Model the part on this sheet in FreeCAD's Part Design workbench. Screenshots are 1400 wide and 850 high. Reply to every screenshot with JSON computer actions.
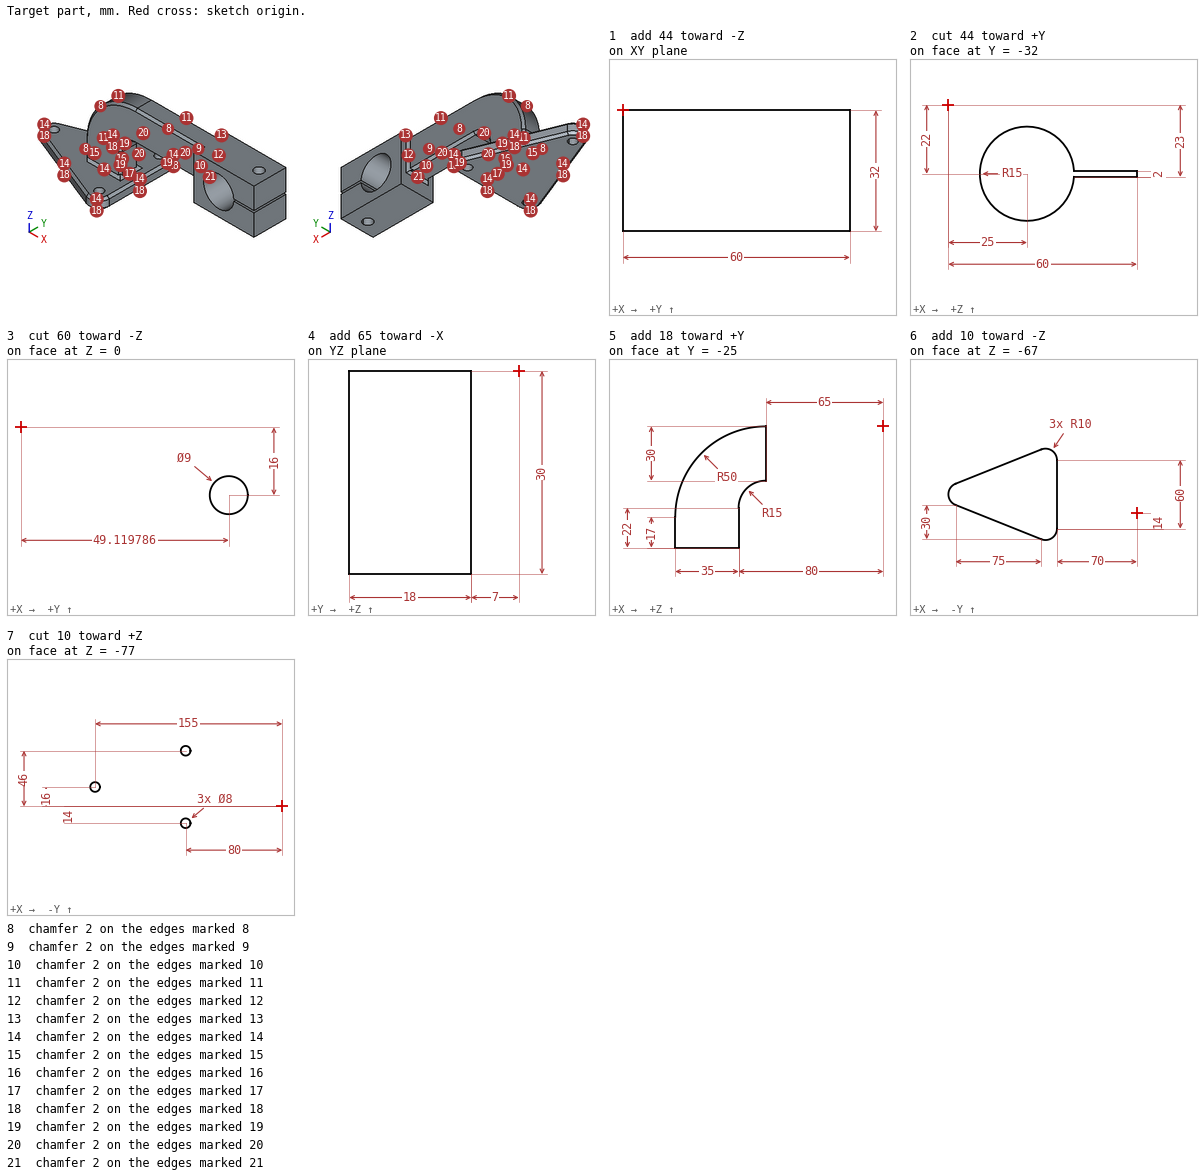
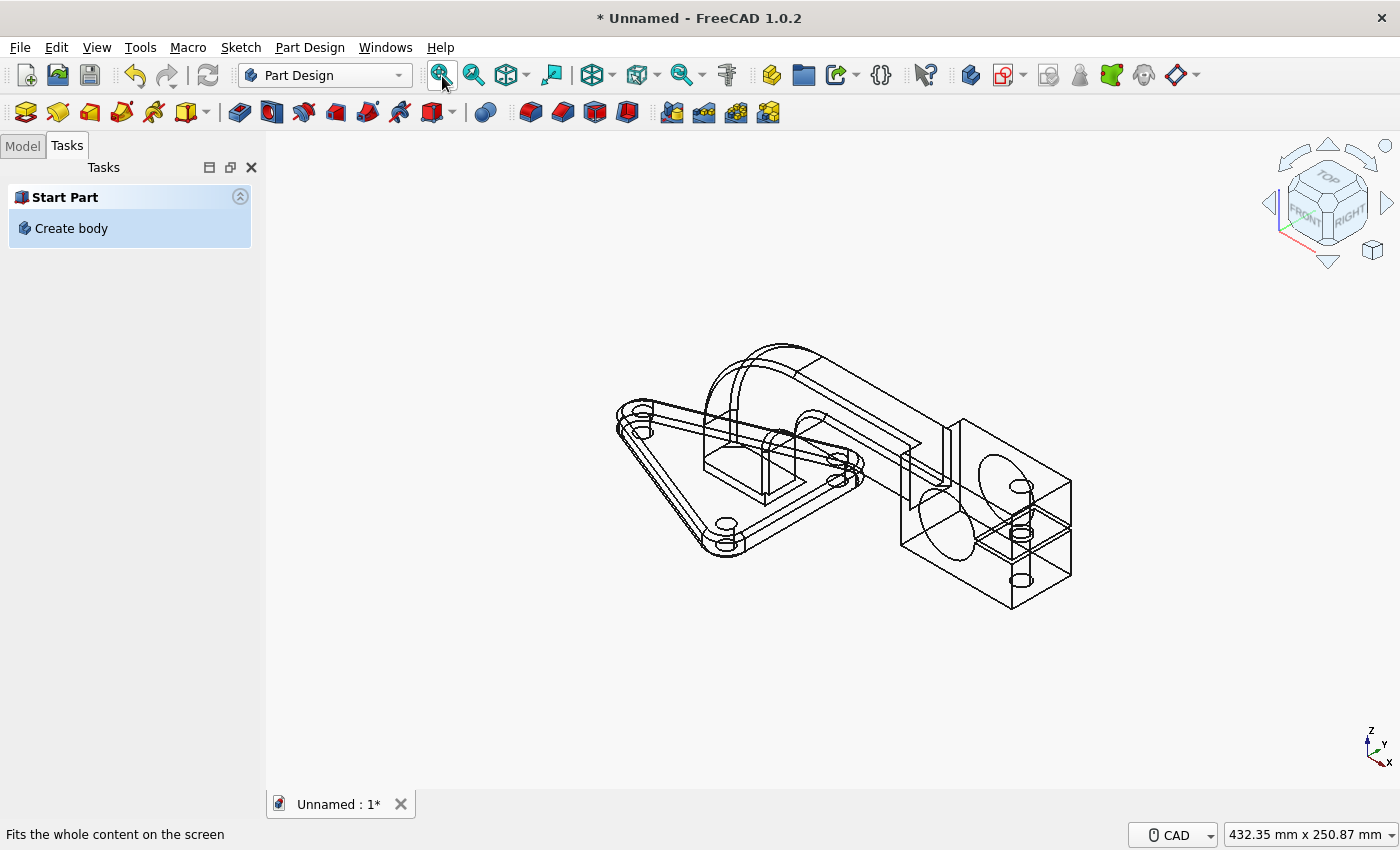
{"action": "left_click", "coordinate": [930, 497]}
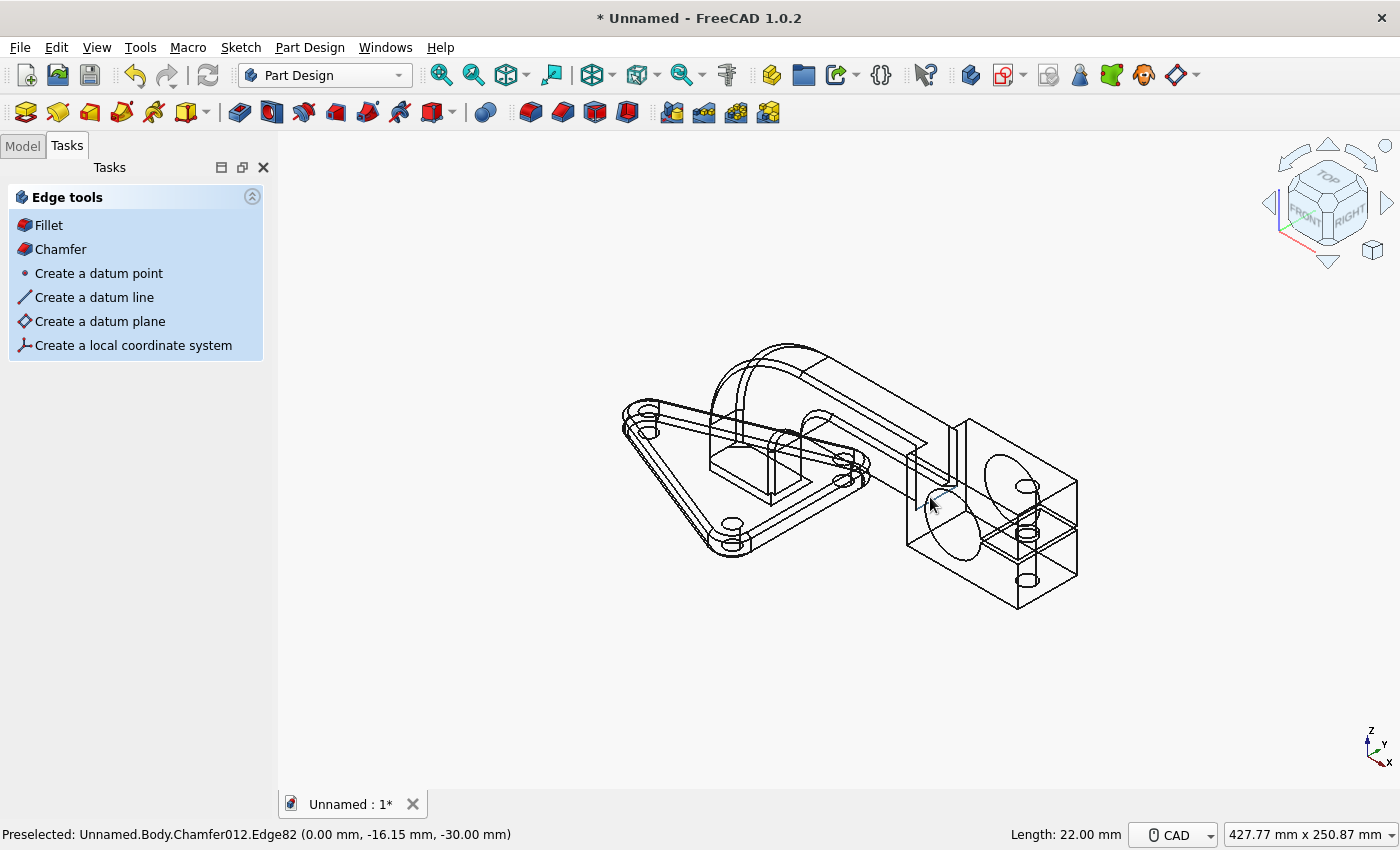
{"action": "key", "text": "v 1"}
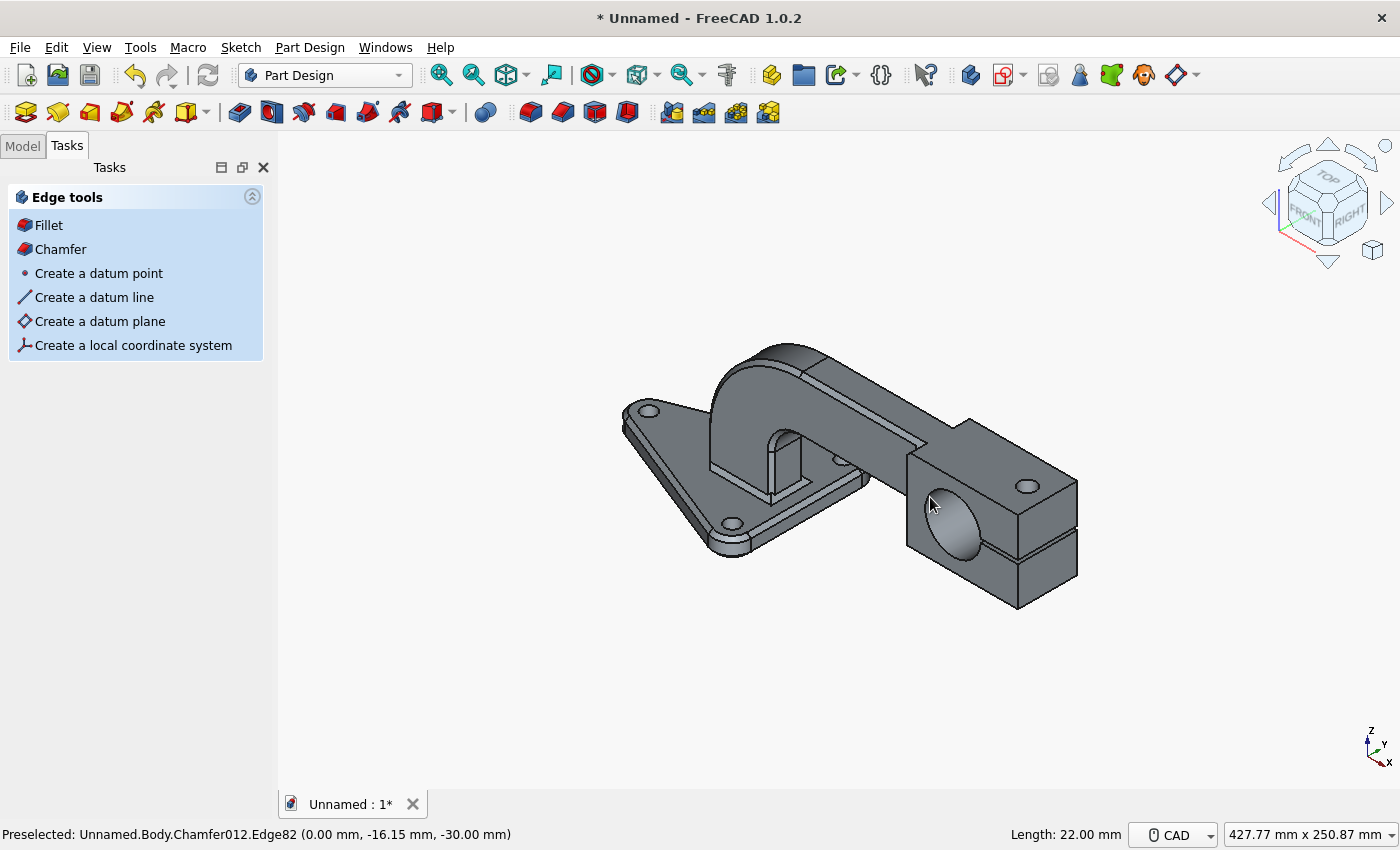
{"action": "left_click", "coordinate": [564, 112]}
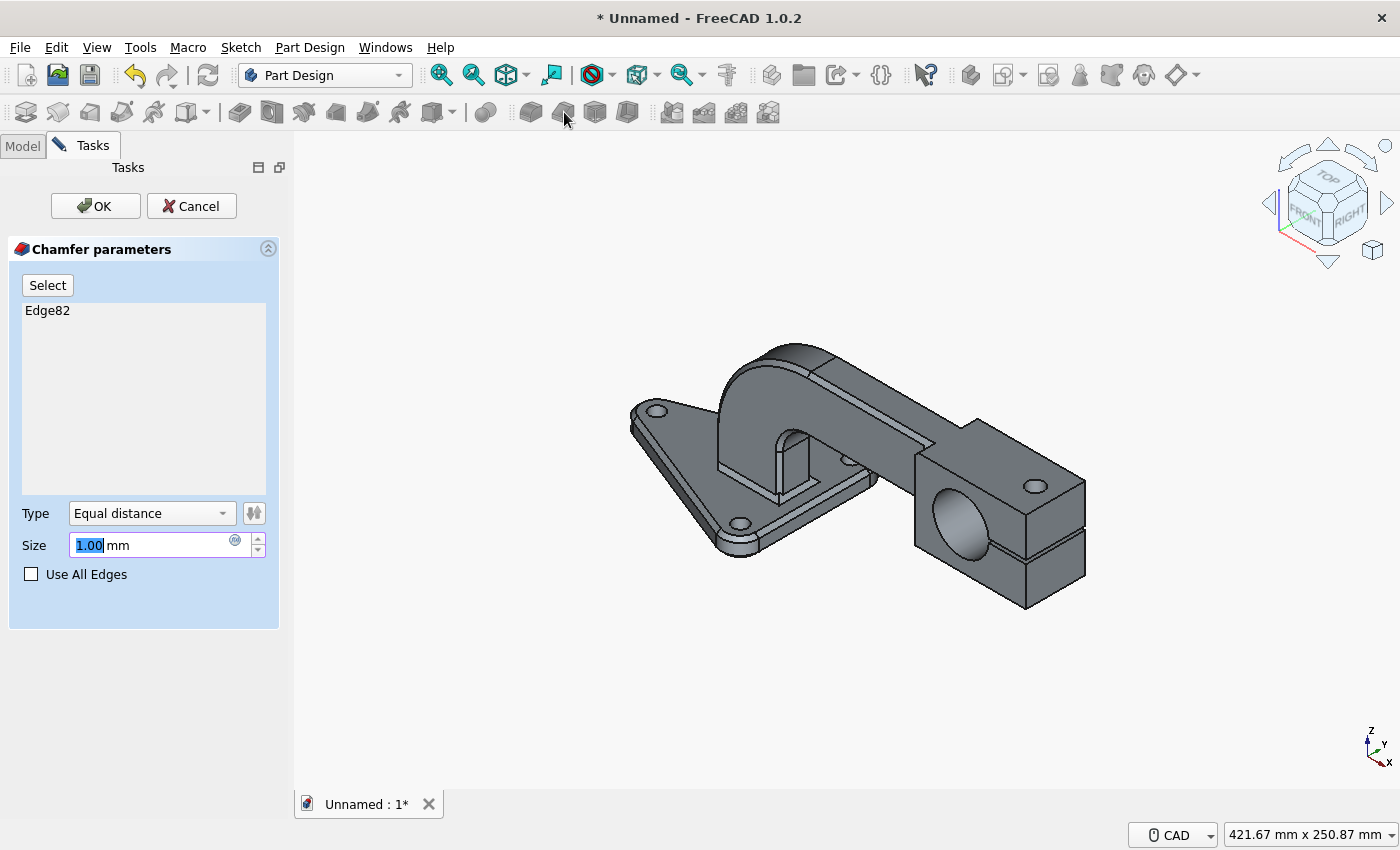
{"action": "type", "text": "2"}
{"action": "key", "text": "Tab"}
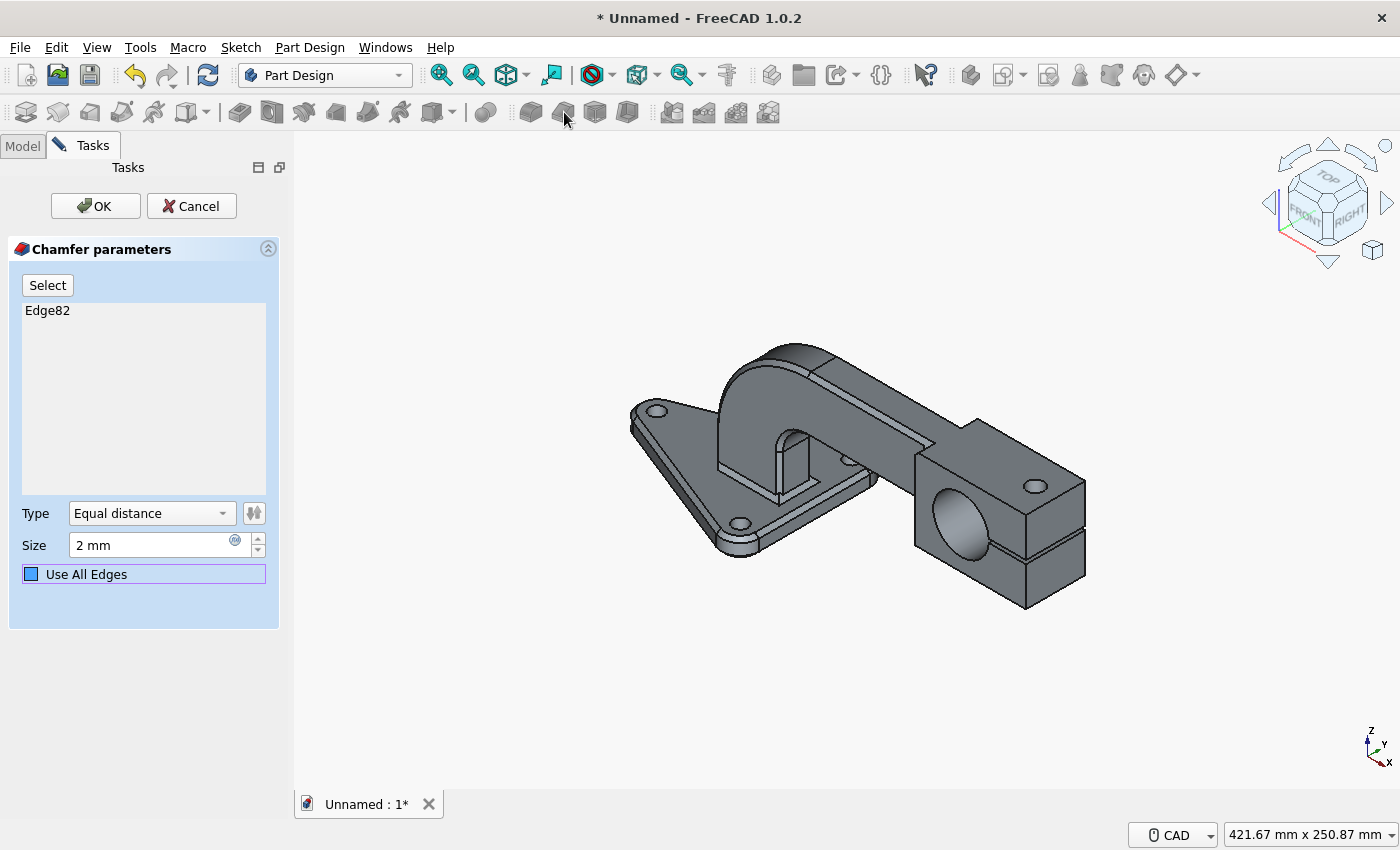
{"action": "left_click", "coordinate": [96, 206]}